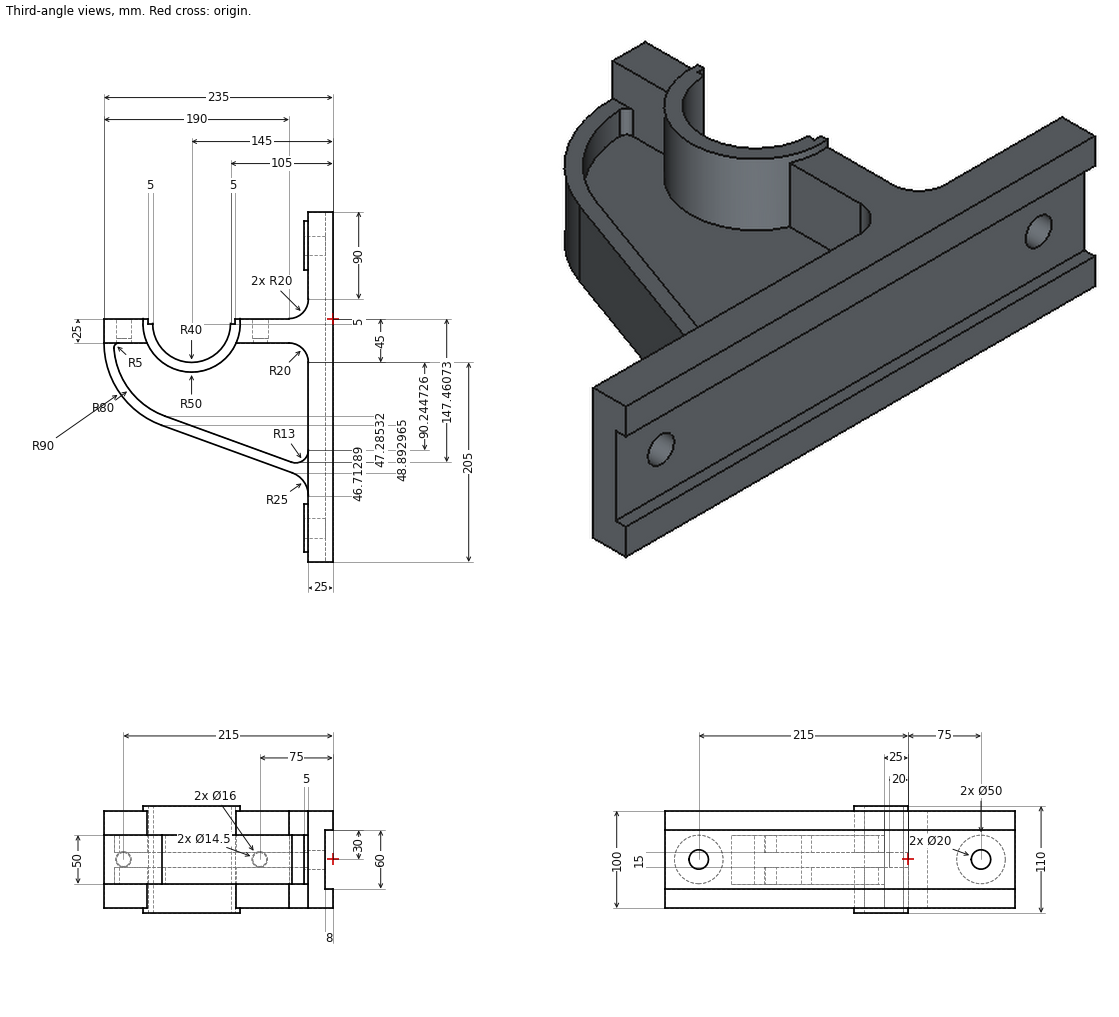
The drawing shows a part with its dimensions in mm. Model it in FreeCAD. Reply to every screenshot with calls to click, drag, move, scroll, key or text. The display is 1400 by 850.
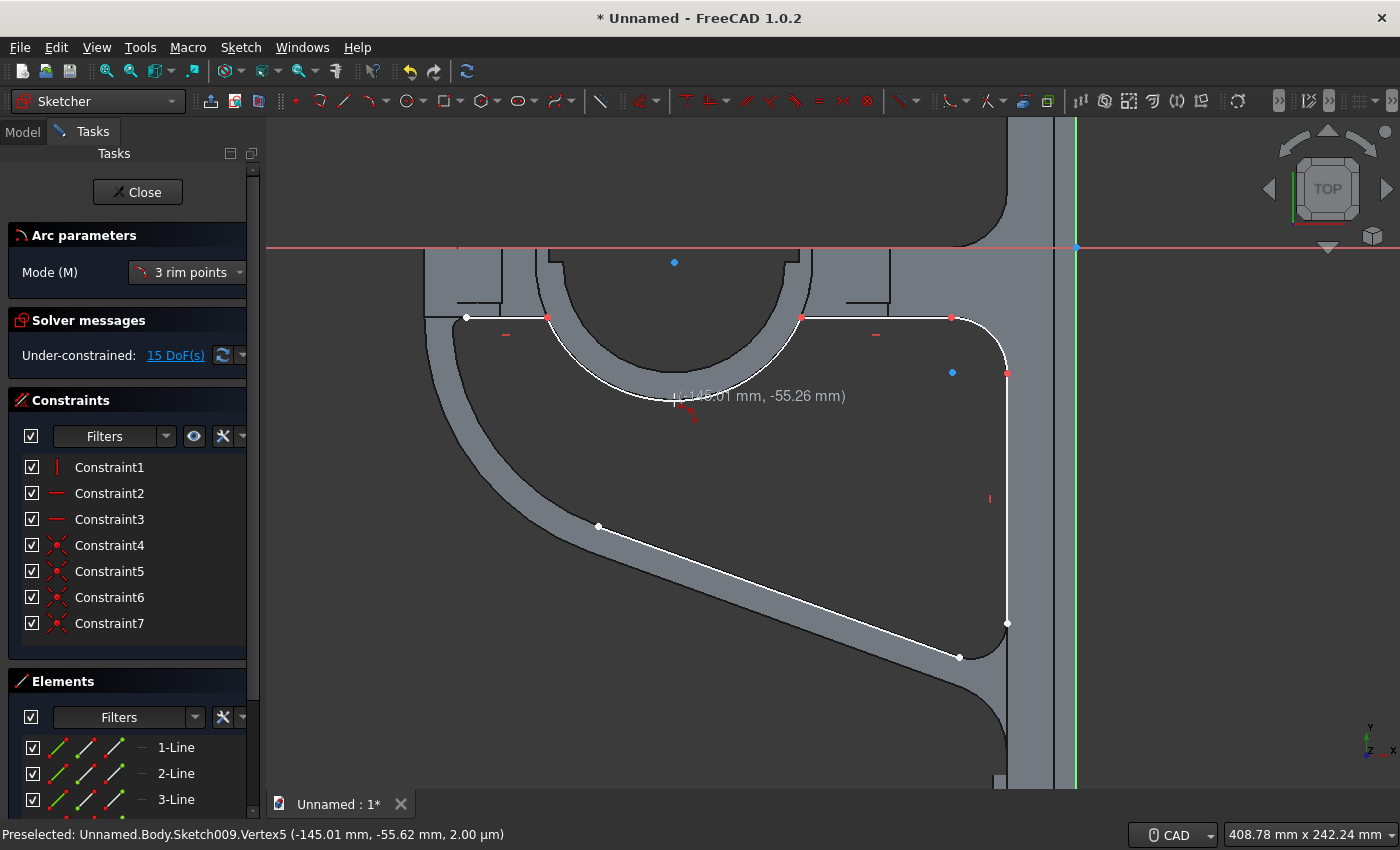
click(466, 318)
click(453, 332)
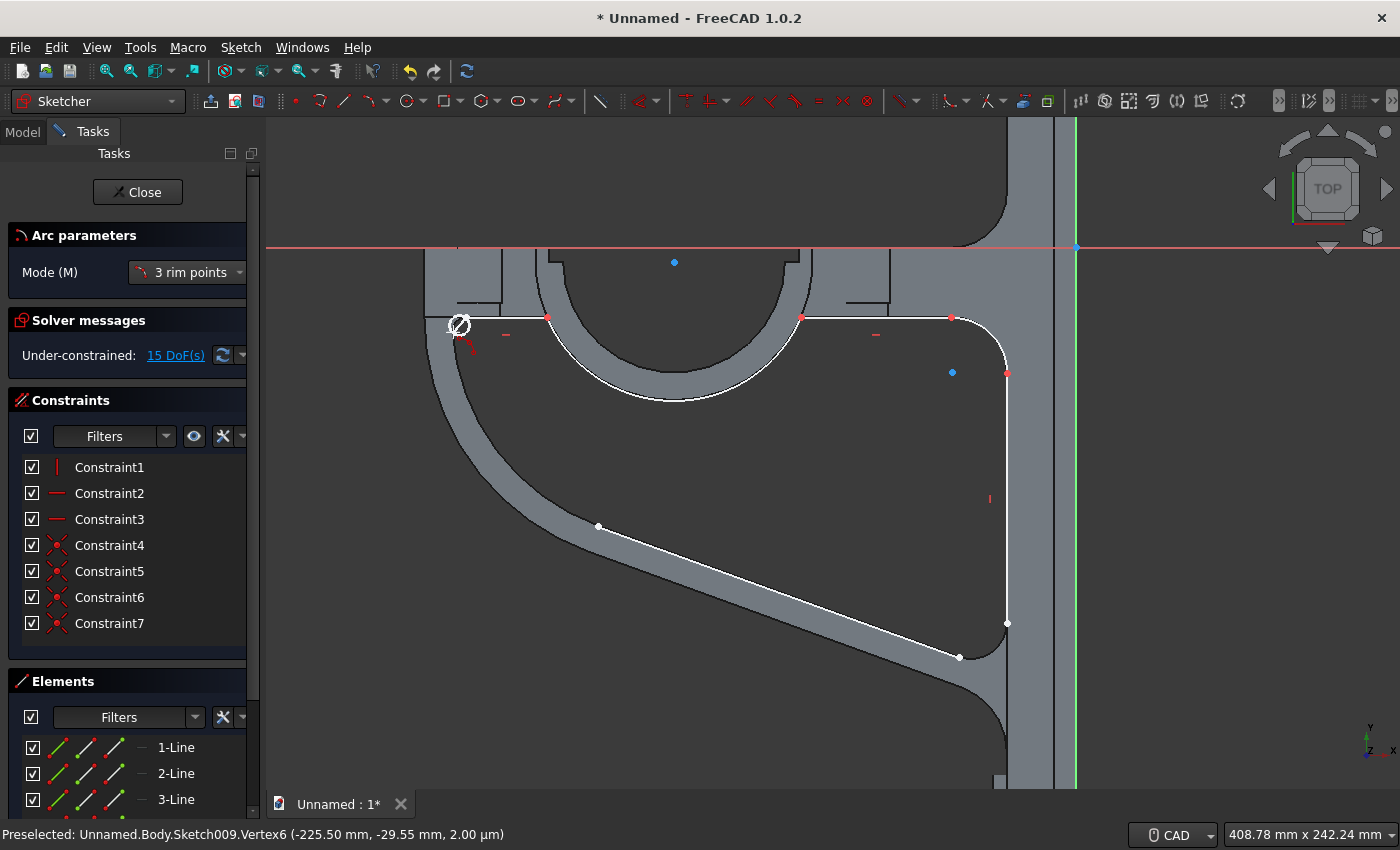
scroll(456, 321, up, 7)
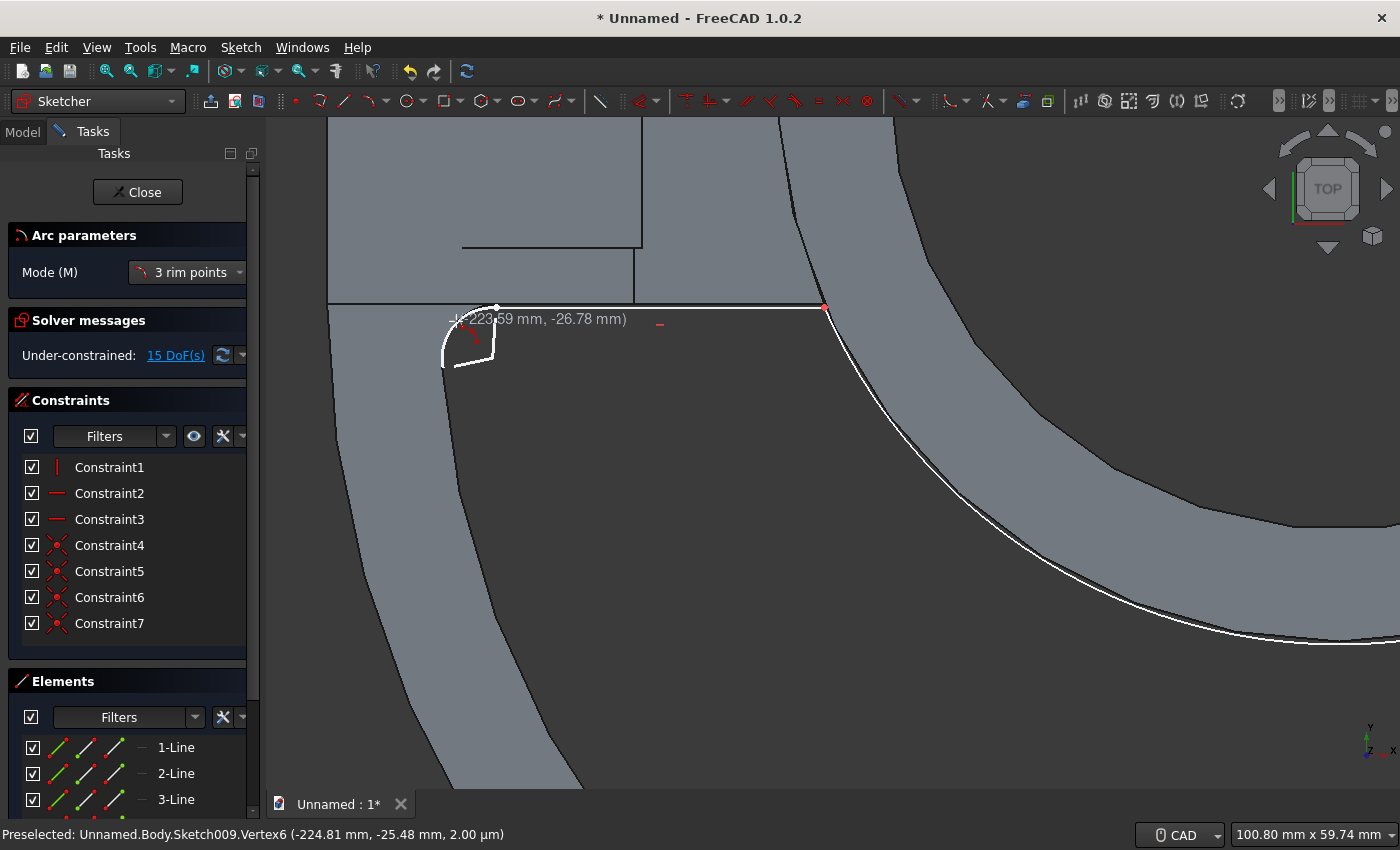
click(457, 322)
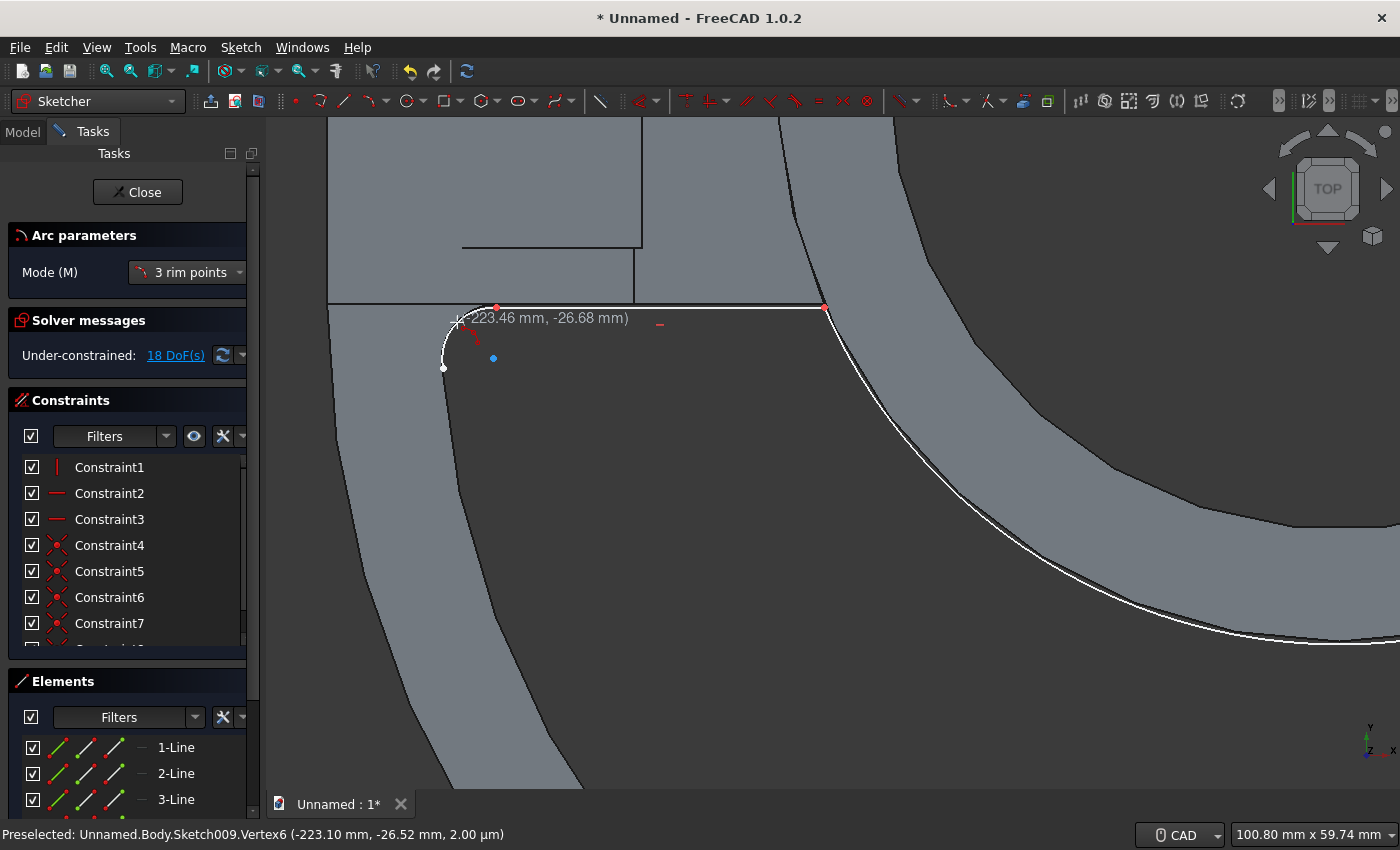
scroll(456, 322, down, 7)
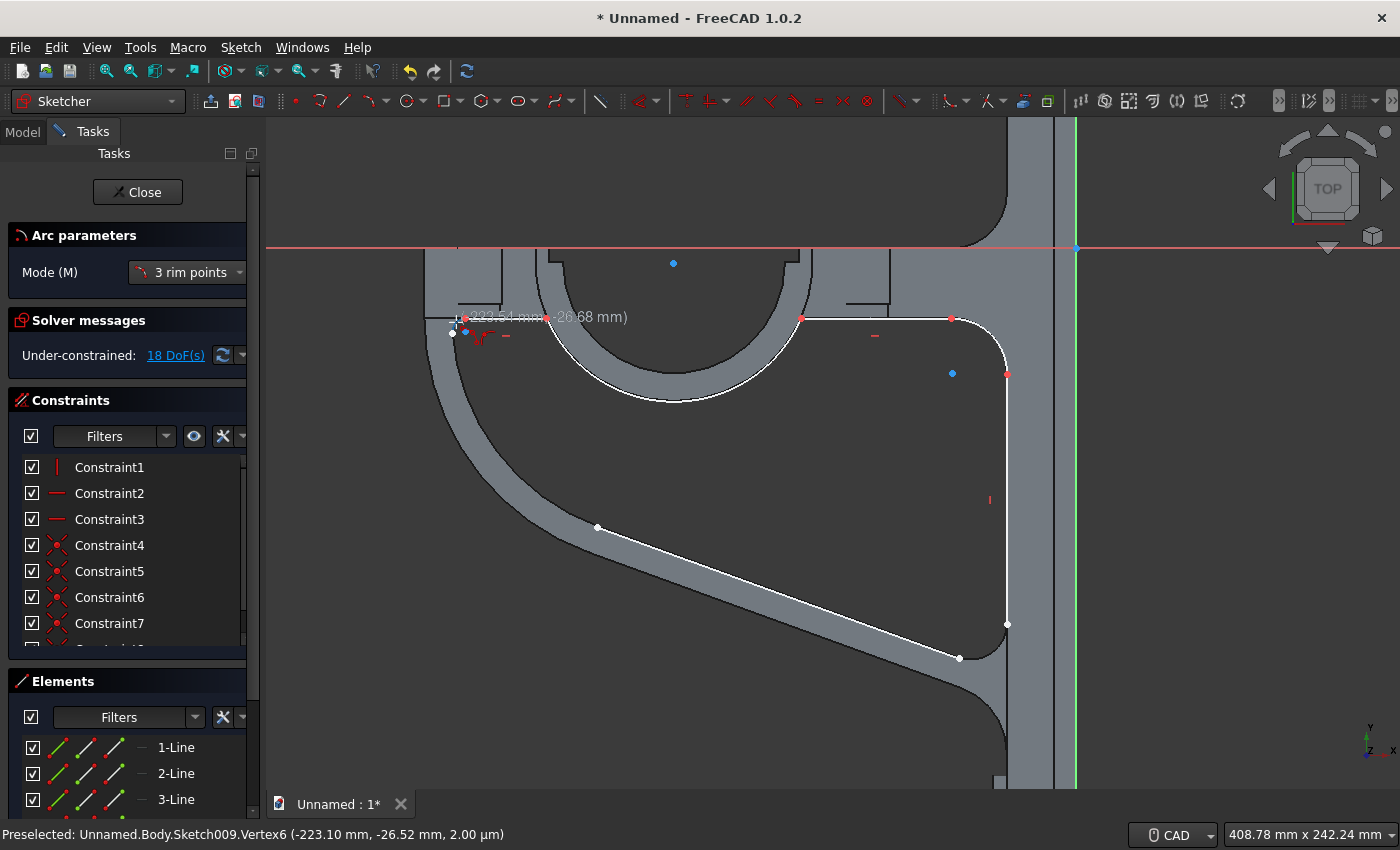
click(453, 334)
click(598, 528)
click(497, 451)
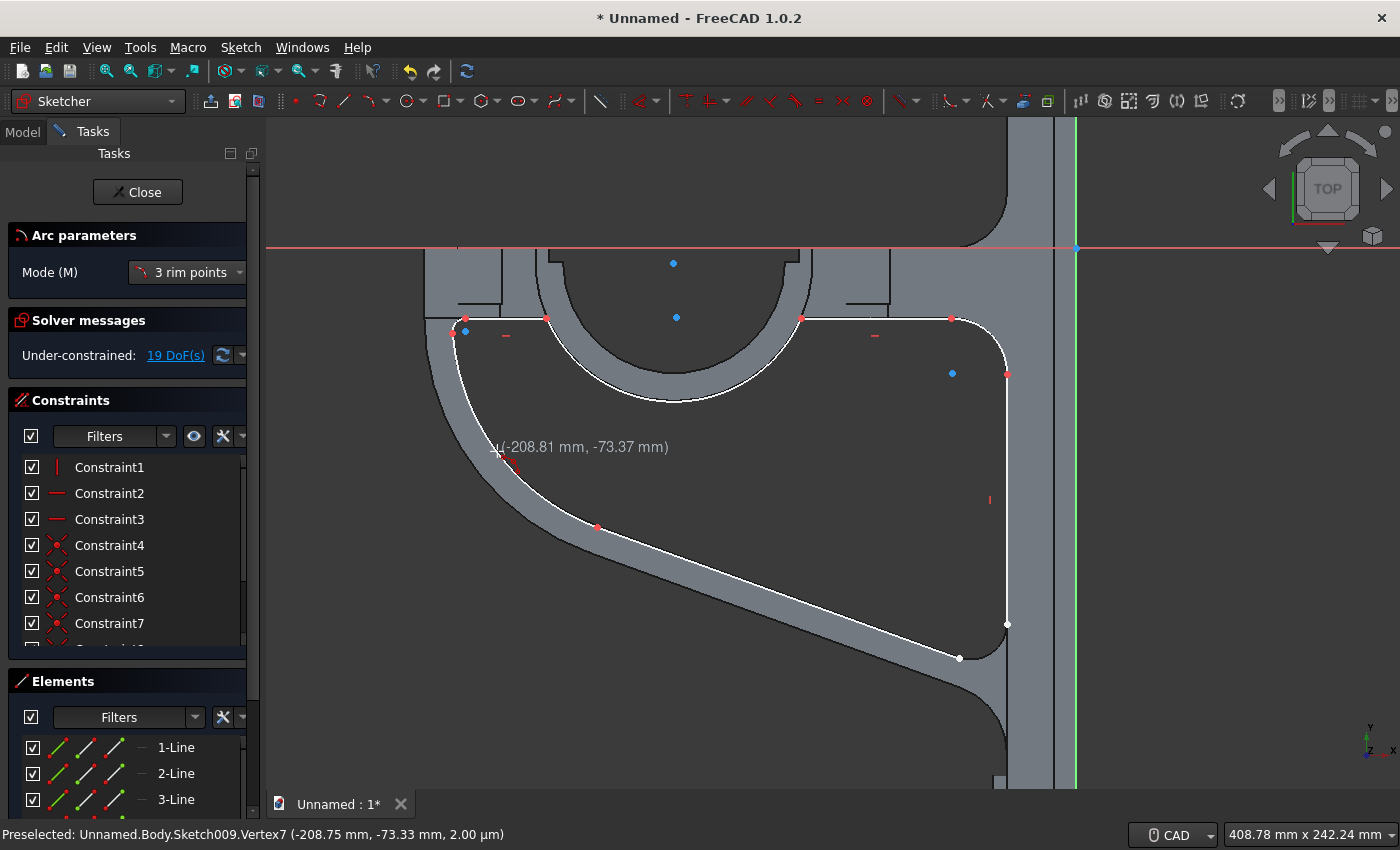
click(959, 659)
click(1007, 625)
click(992, 653)
key(Escape)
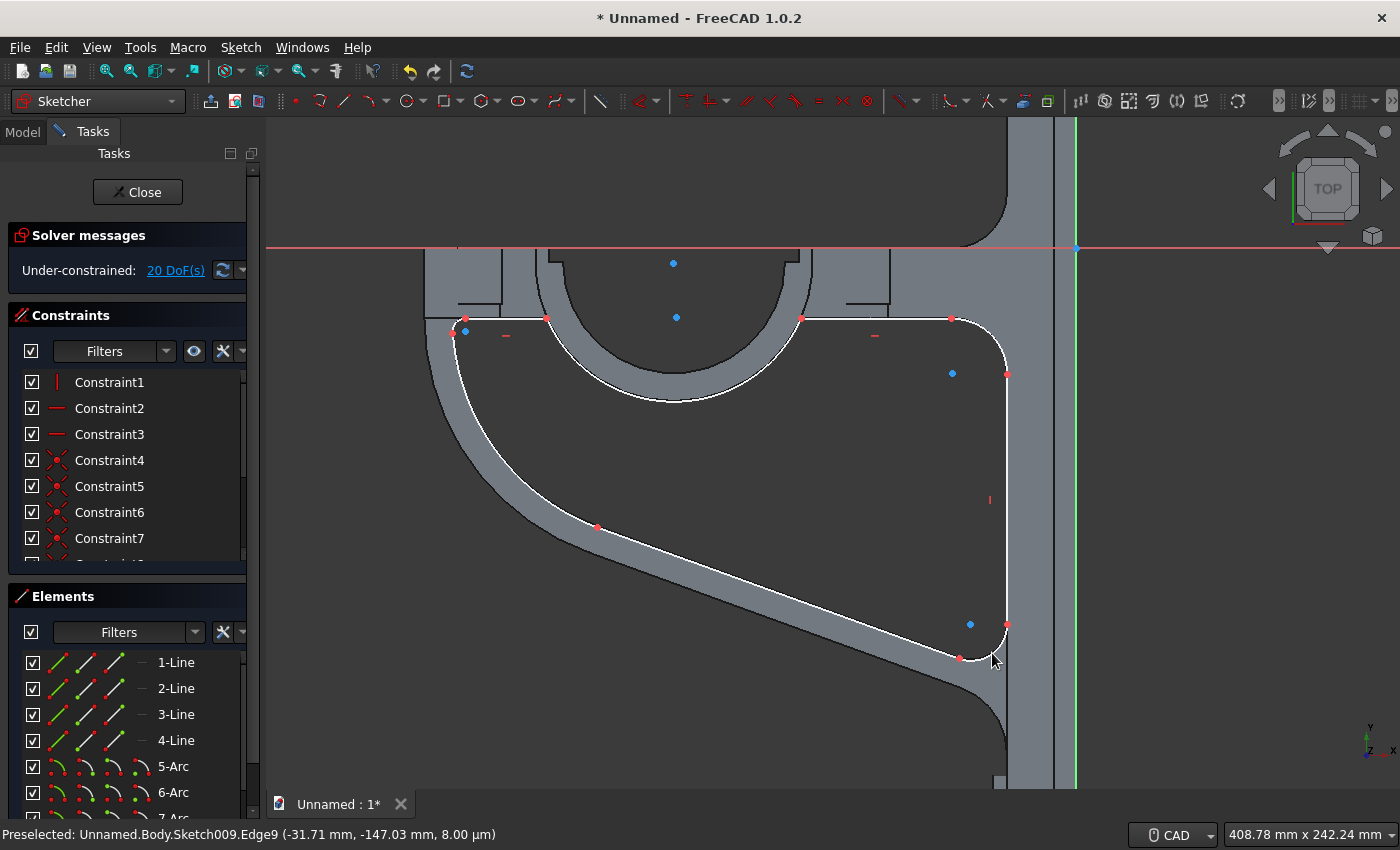
click(1007, 550)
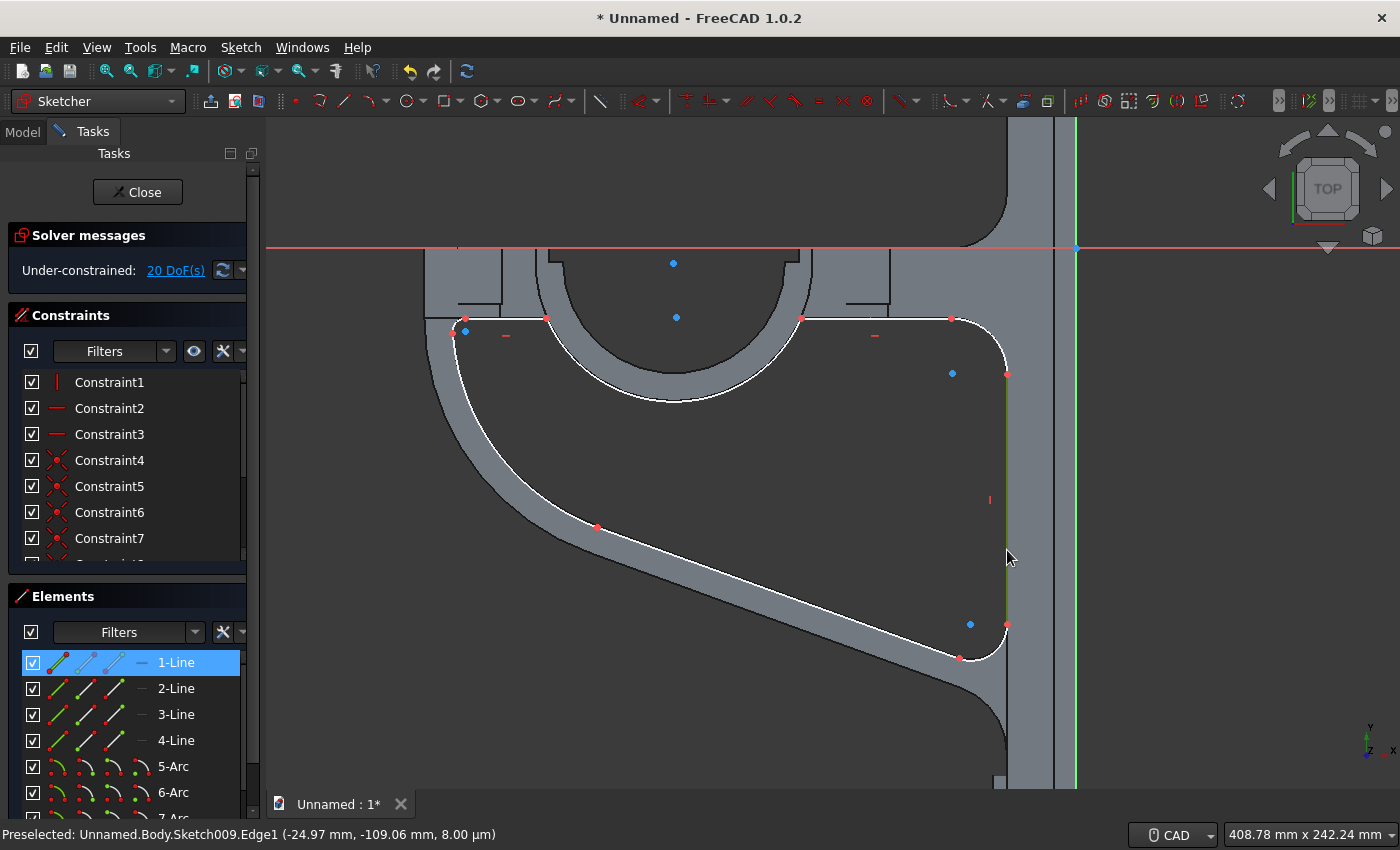
click(1001, 349)